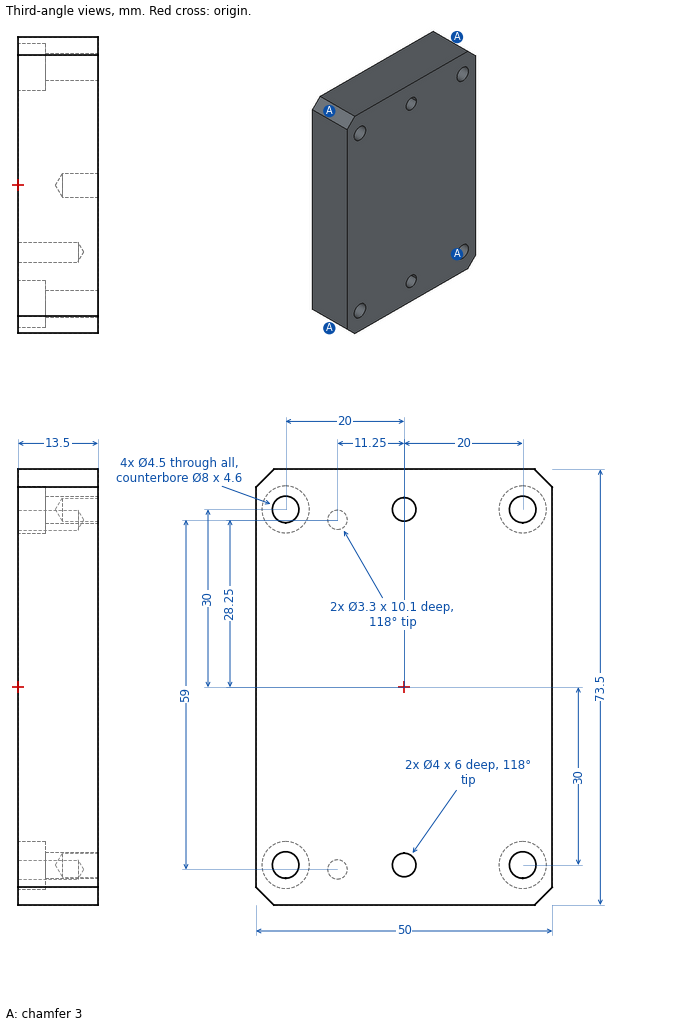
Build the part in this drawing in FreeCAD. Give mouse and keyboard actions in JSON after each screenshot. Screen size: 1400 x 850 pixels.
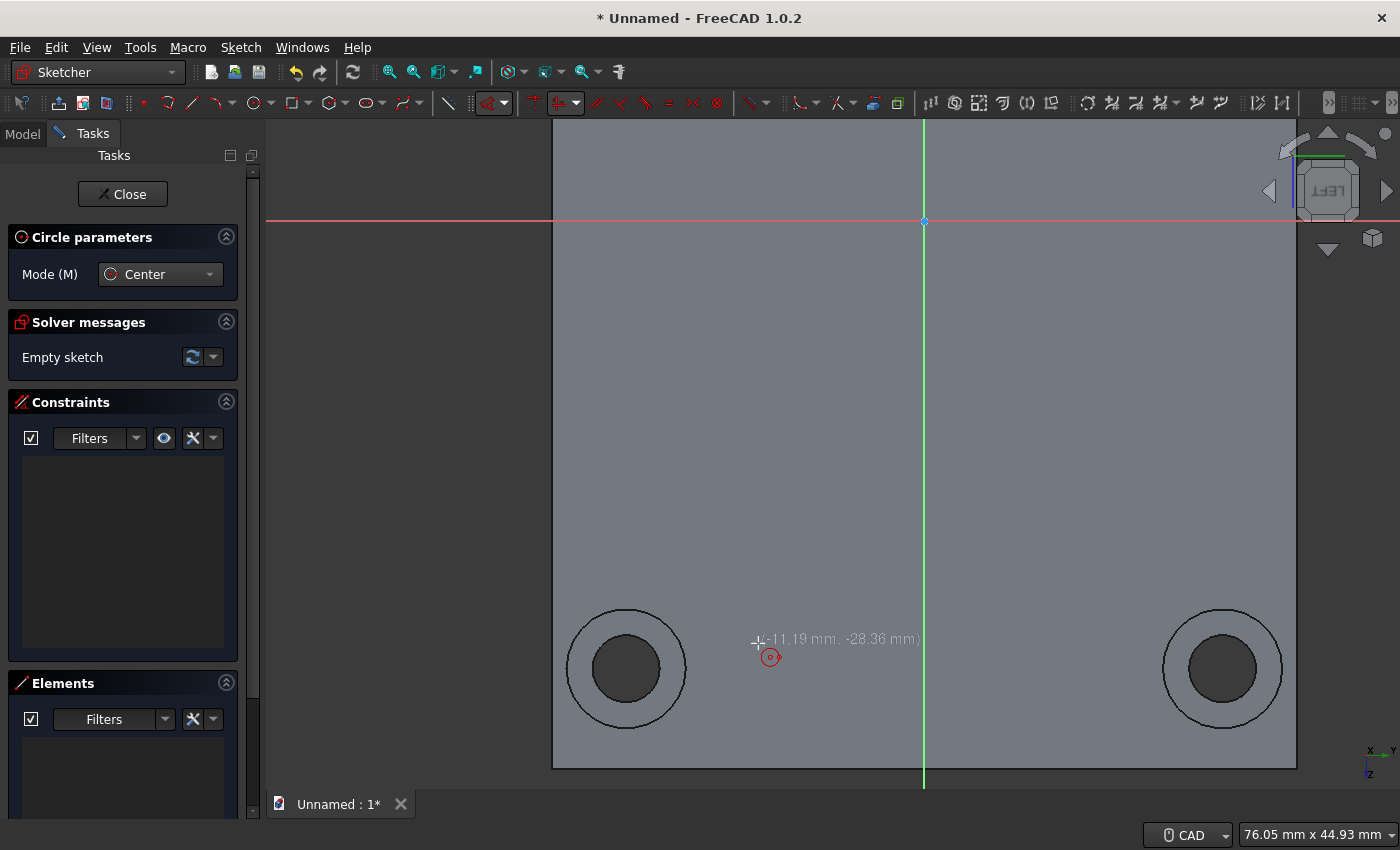
{"action": "left_click", "coordinate": [757, 643]}
{"action": "mouse_move", "coordinate": [774, 625]}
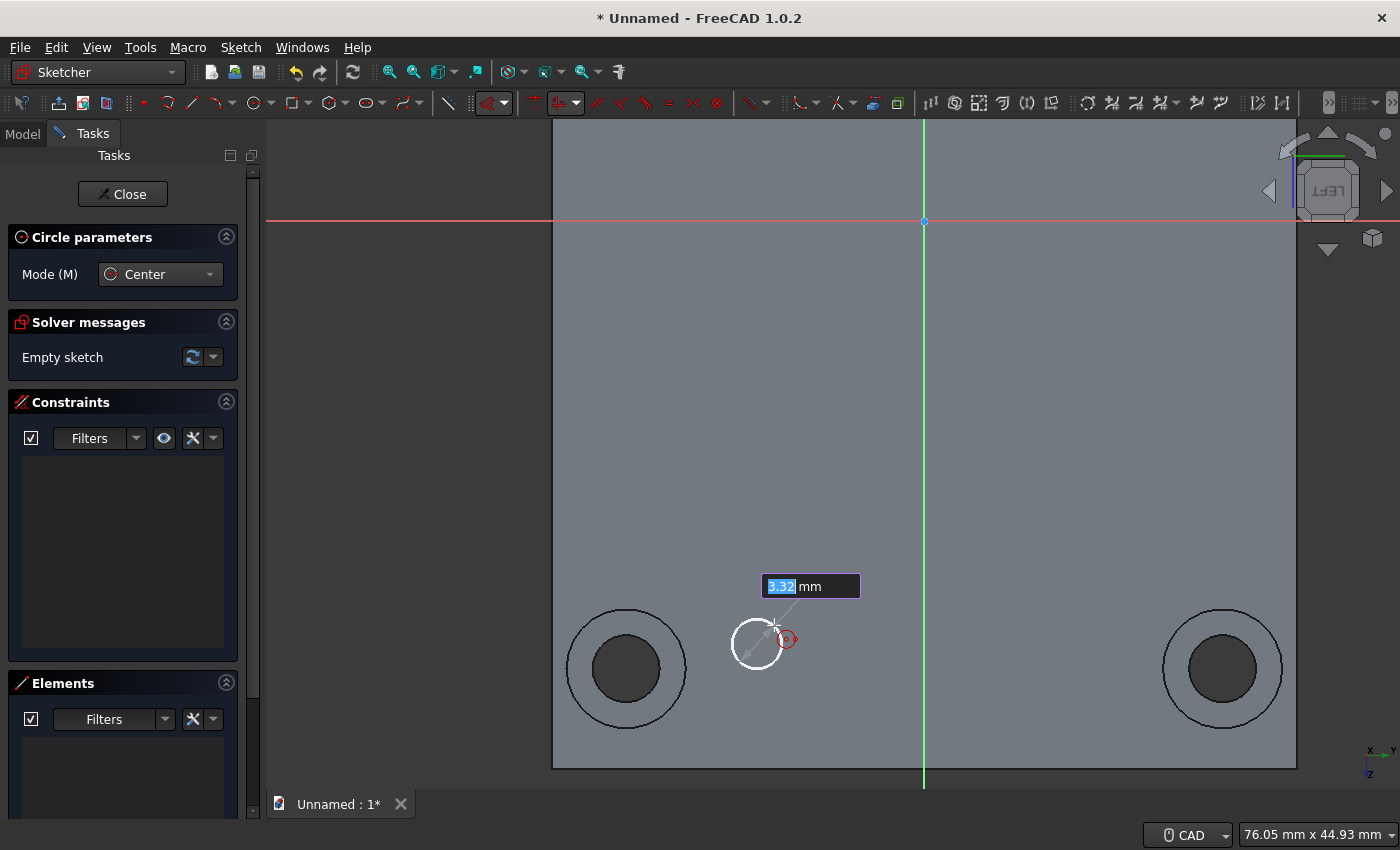
{"action": "type", "text": "3.3"}
{"action": "key", "text": "Return"}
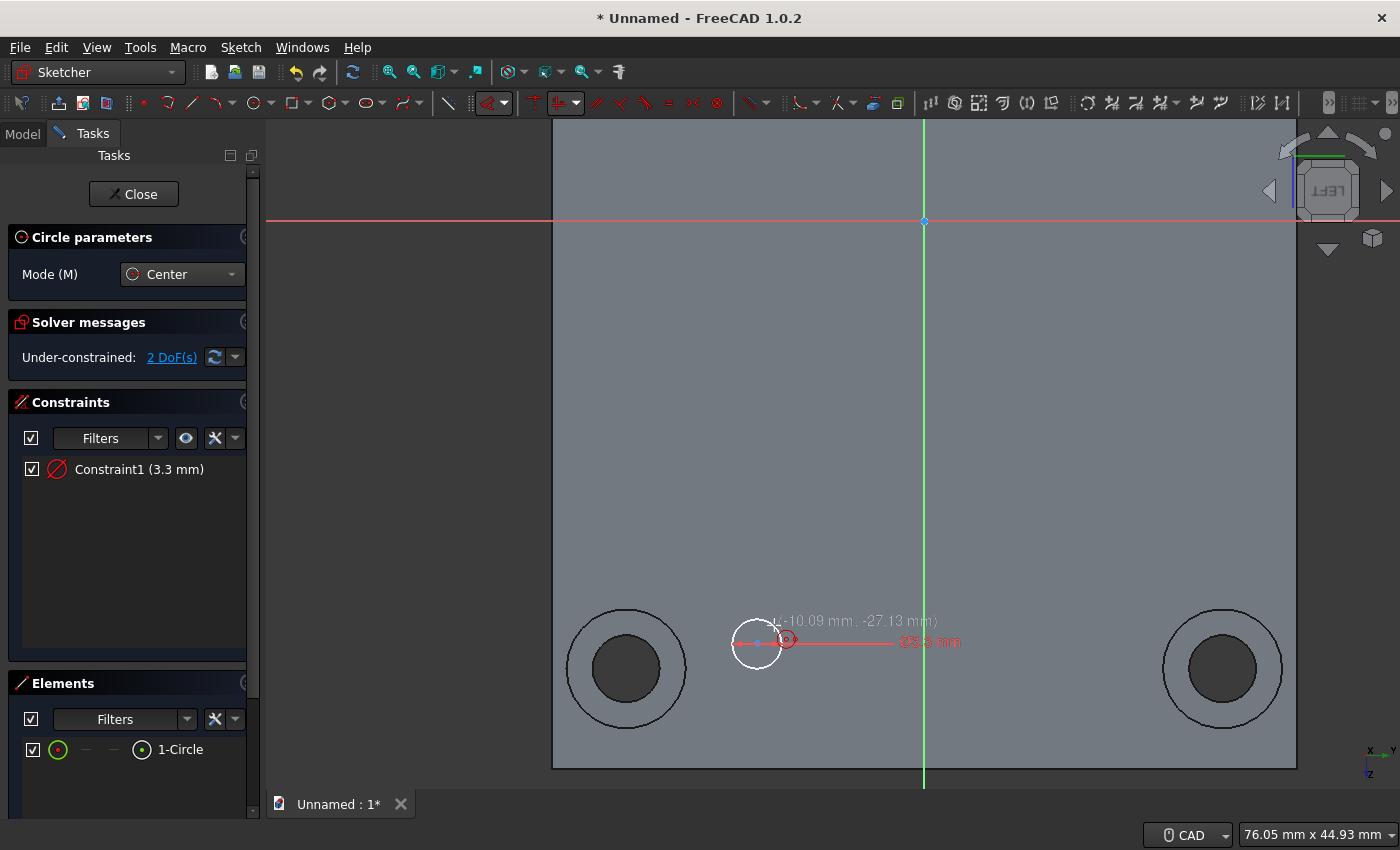
{"action": "scroll", "coordinate": [713, 659], "scroll_direction": "down", "scroll_amount": 4}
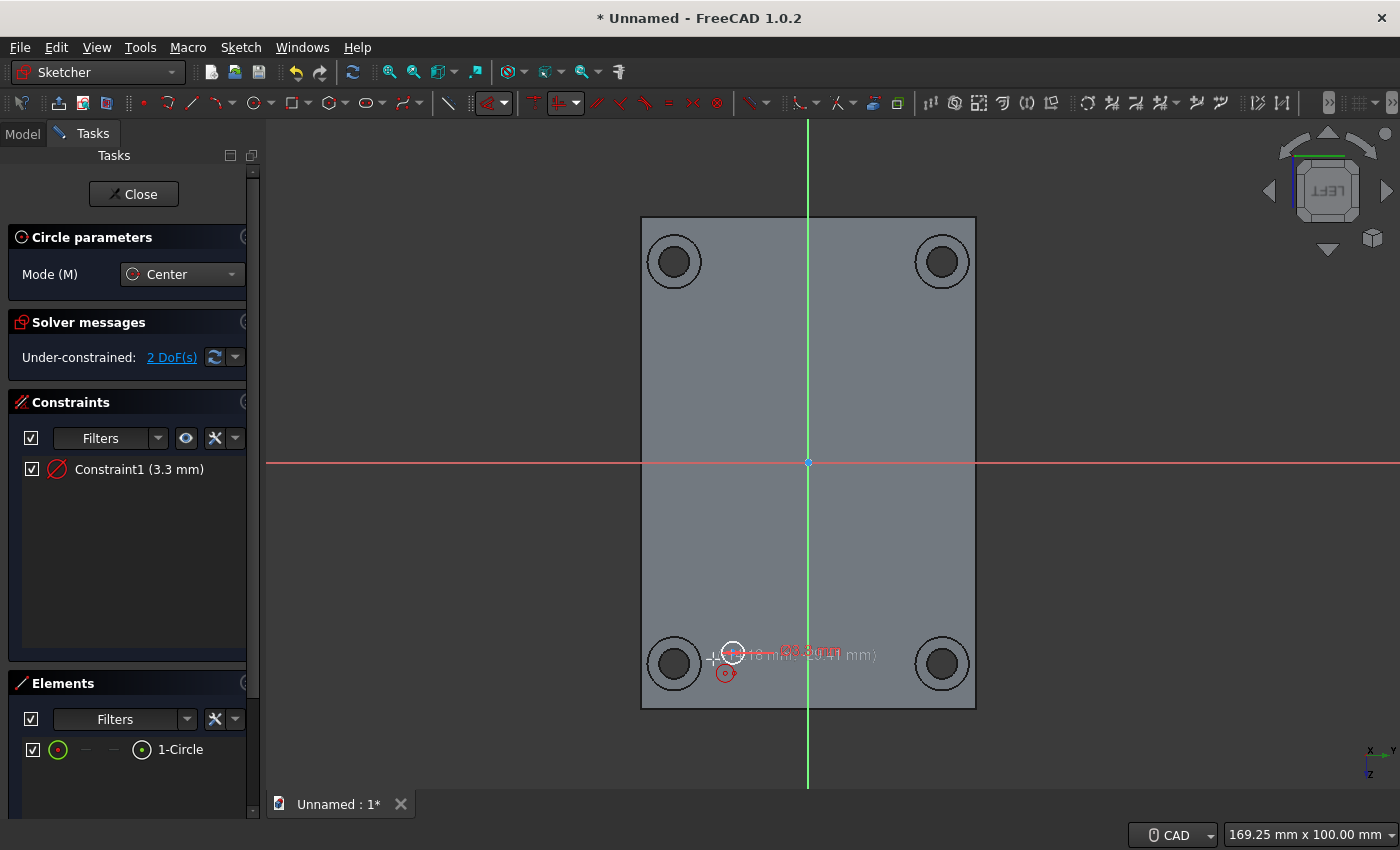
{"action": "scroll", "coordinate": [733, 257], "scroll_direction": "up", "scroll_amount": 4}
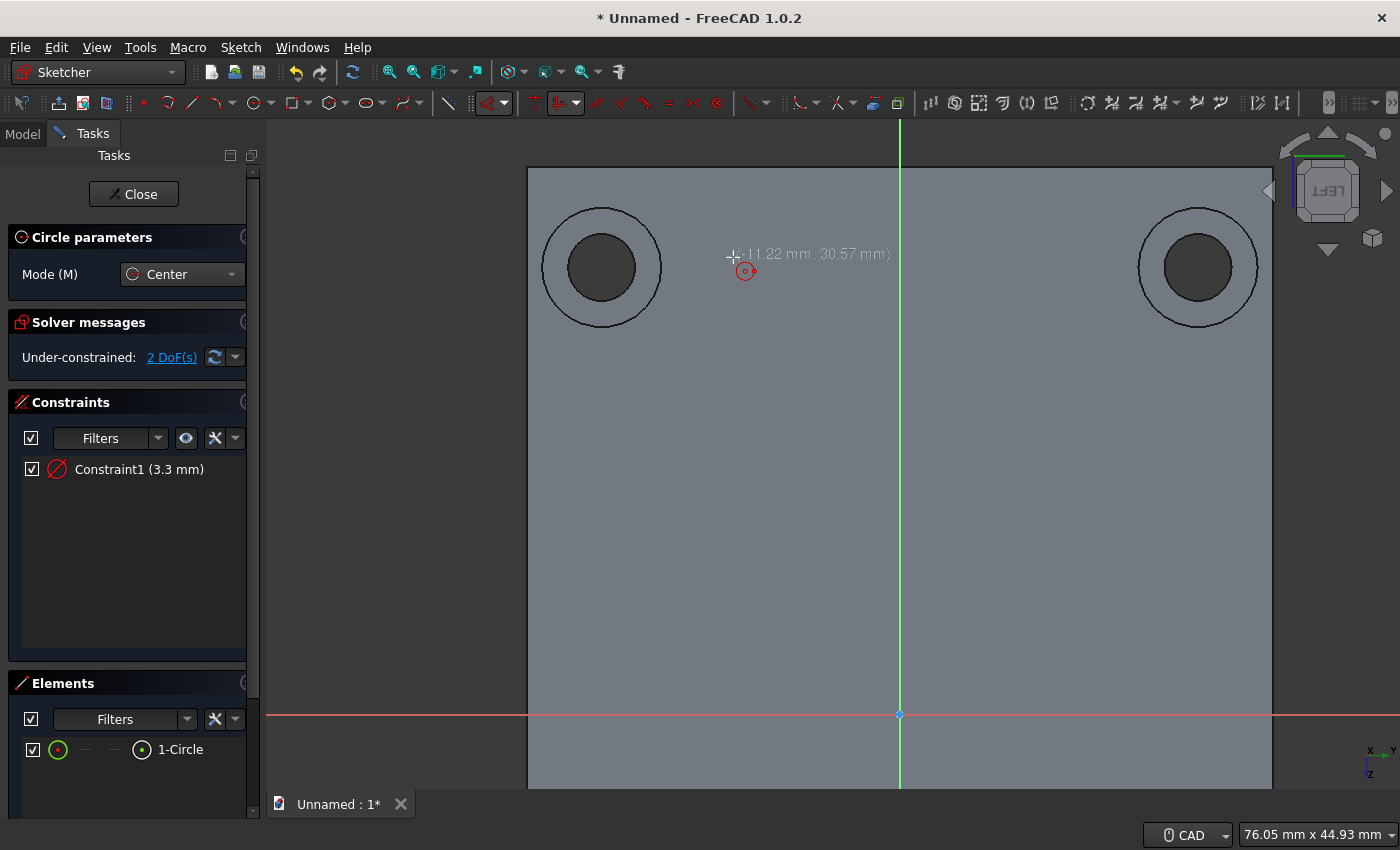
{"action": "left_click", "coordinate": [732, 256]}
{"action": "mouse_move", "coordinate": [749, 239]}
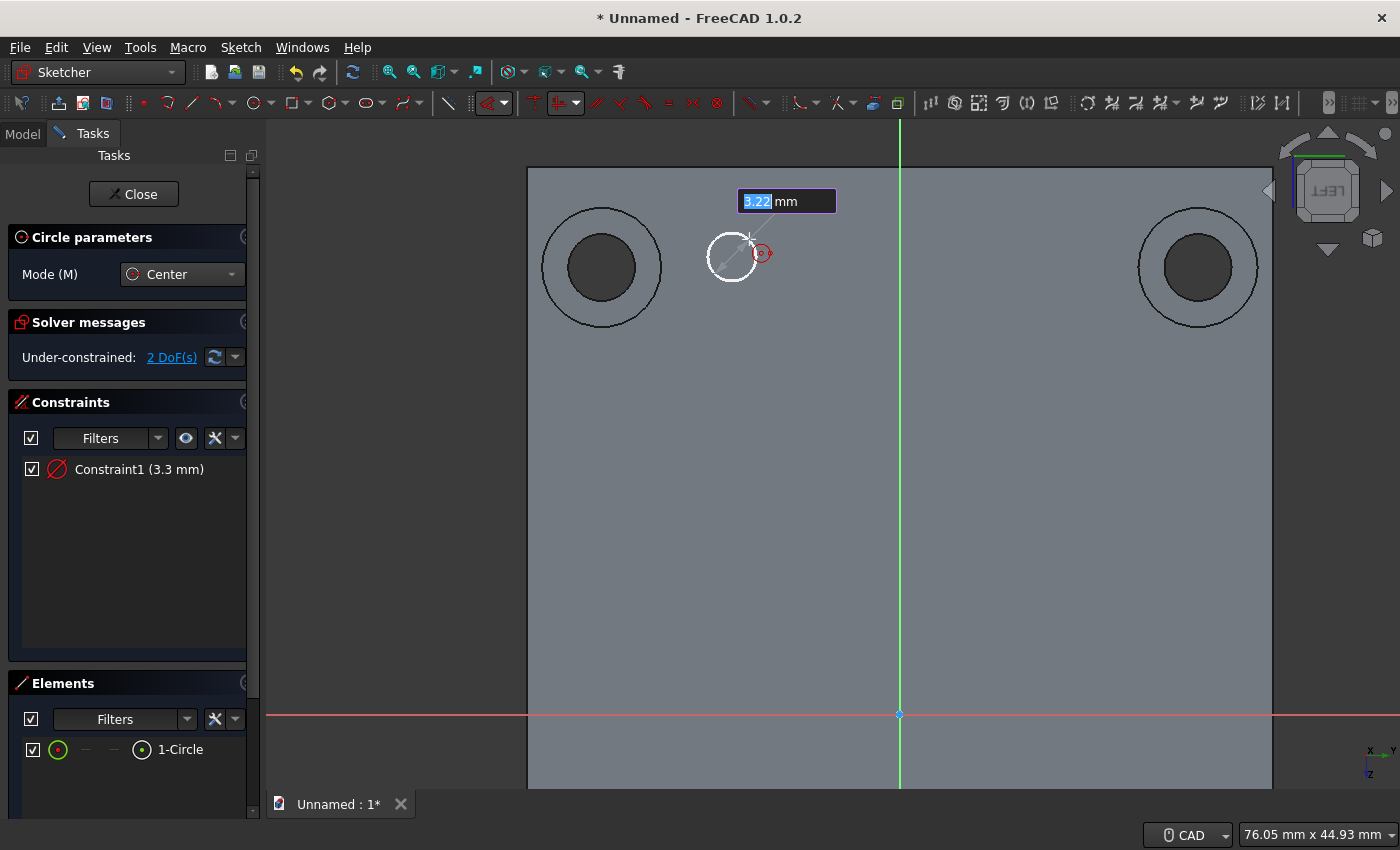
{"action": "type", "text": "3.3"}
{"action": "key", "text": "Return"}
{"action": "key", "text": "Escape"}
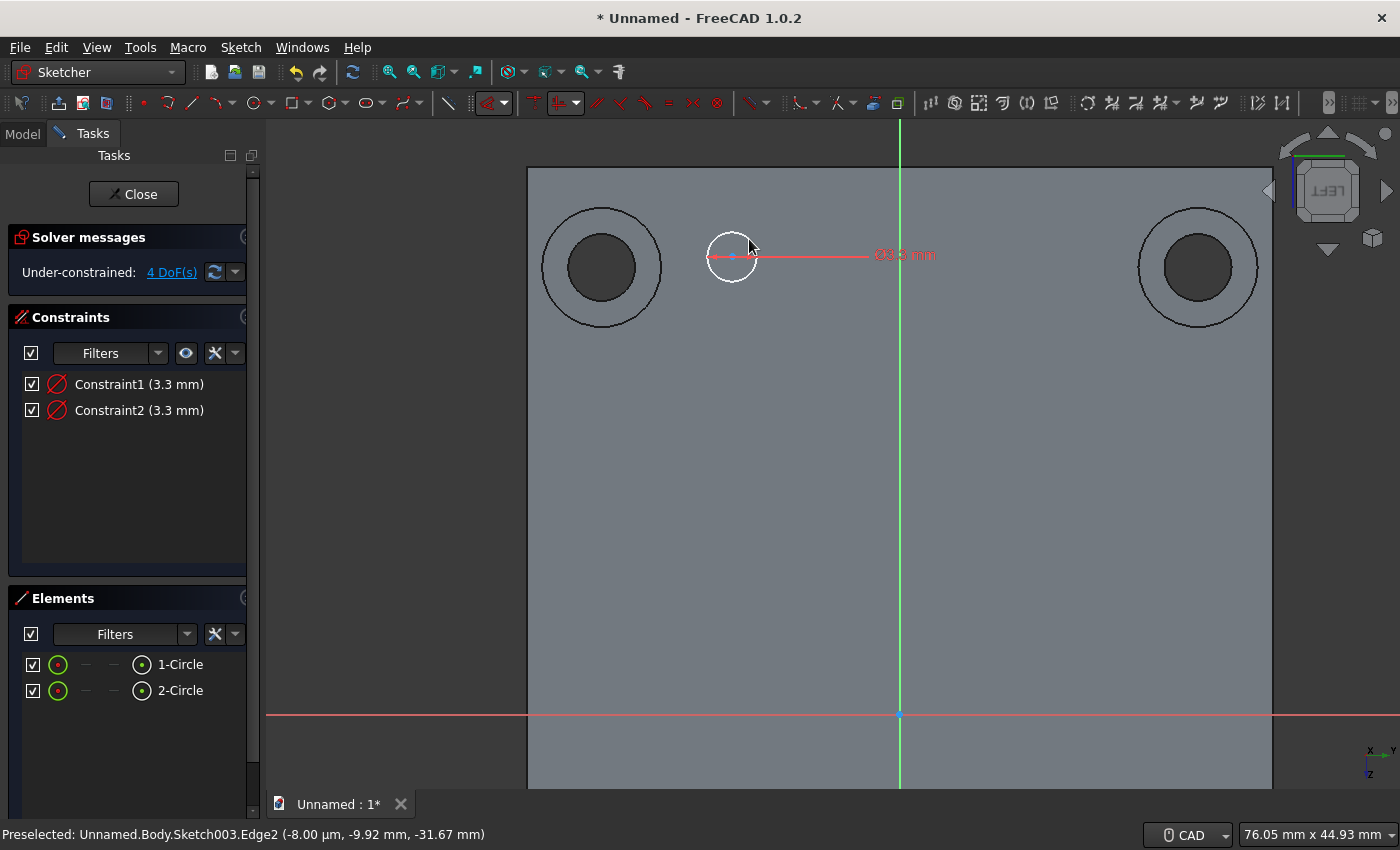
{"action": "scroll", "coordinate": [733, 256], "scroll_direction": "down", "scroll_amount": 4}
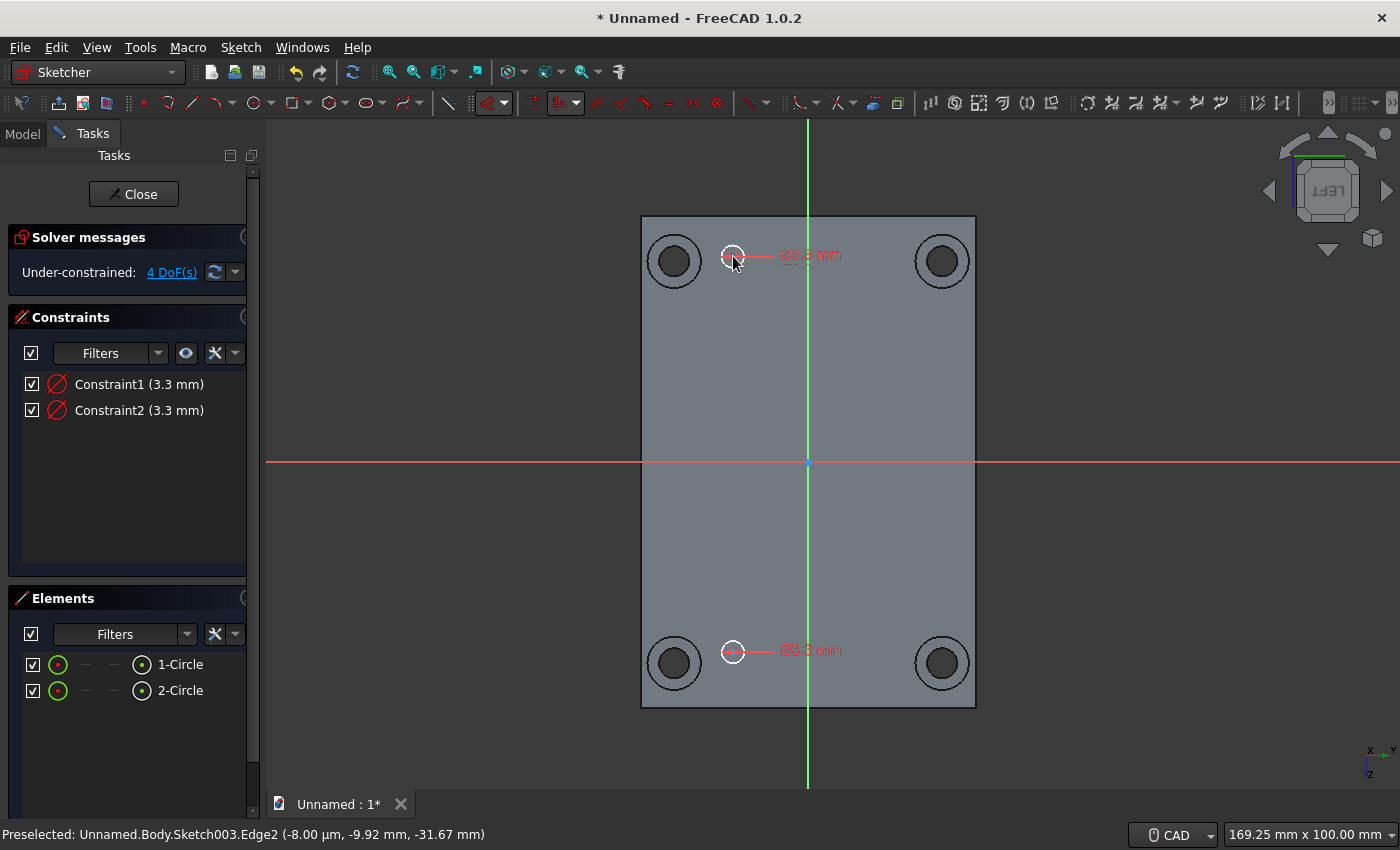
{"action": "left_click", "coordinate": [733, 652]}